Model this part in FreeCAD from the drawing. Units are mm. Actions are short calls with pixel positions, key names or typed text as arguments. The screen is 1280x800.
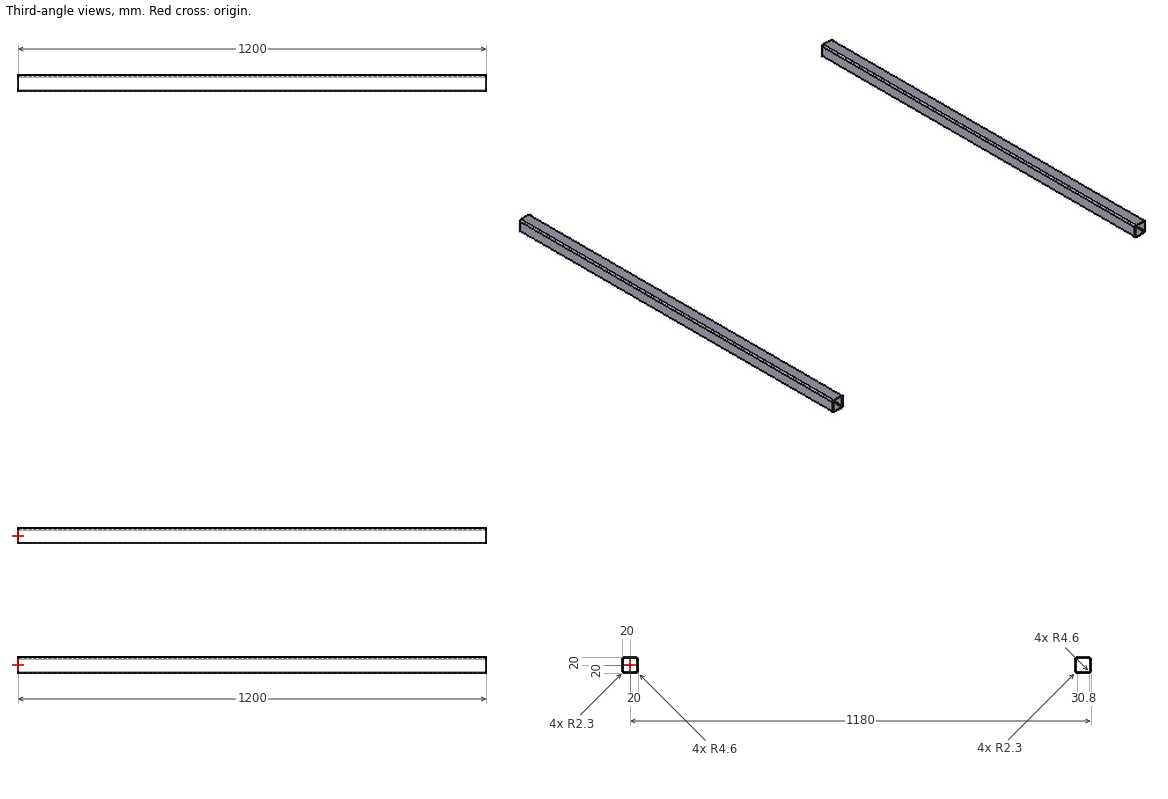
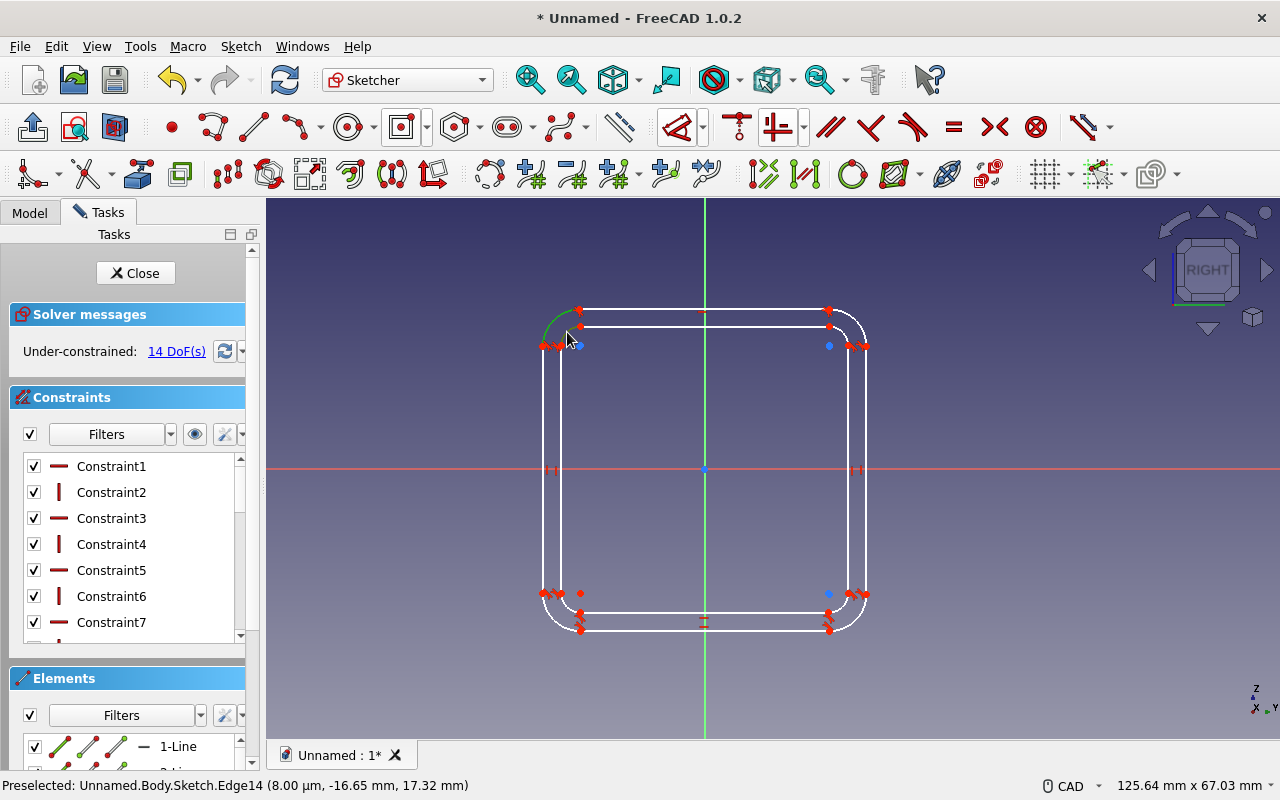
key(c)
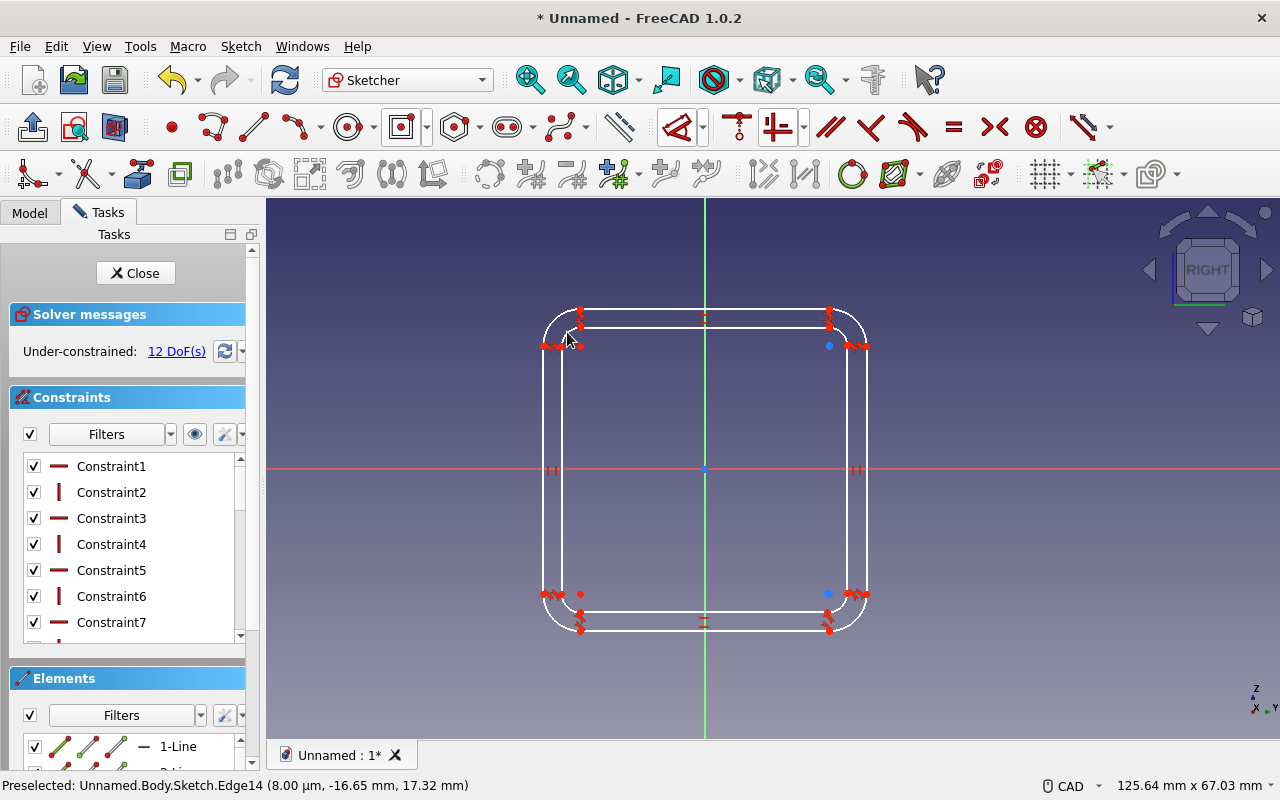
click(863, 329)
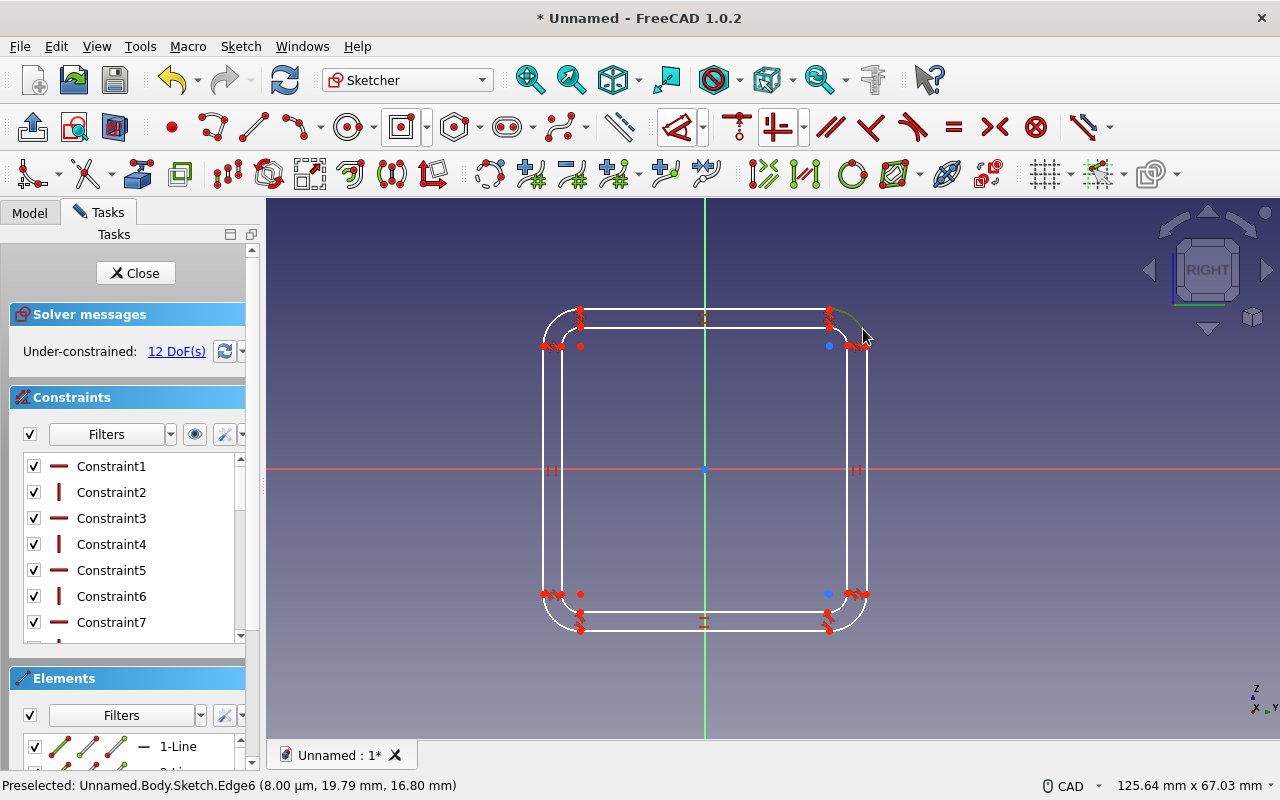
click(842, 333)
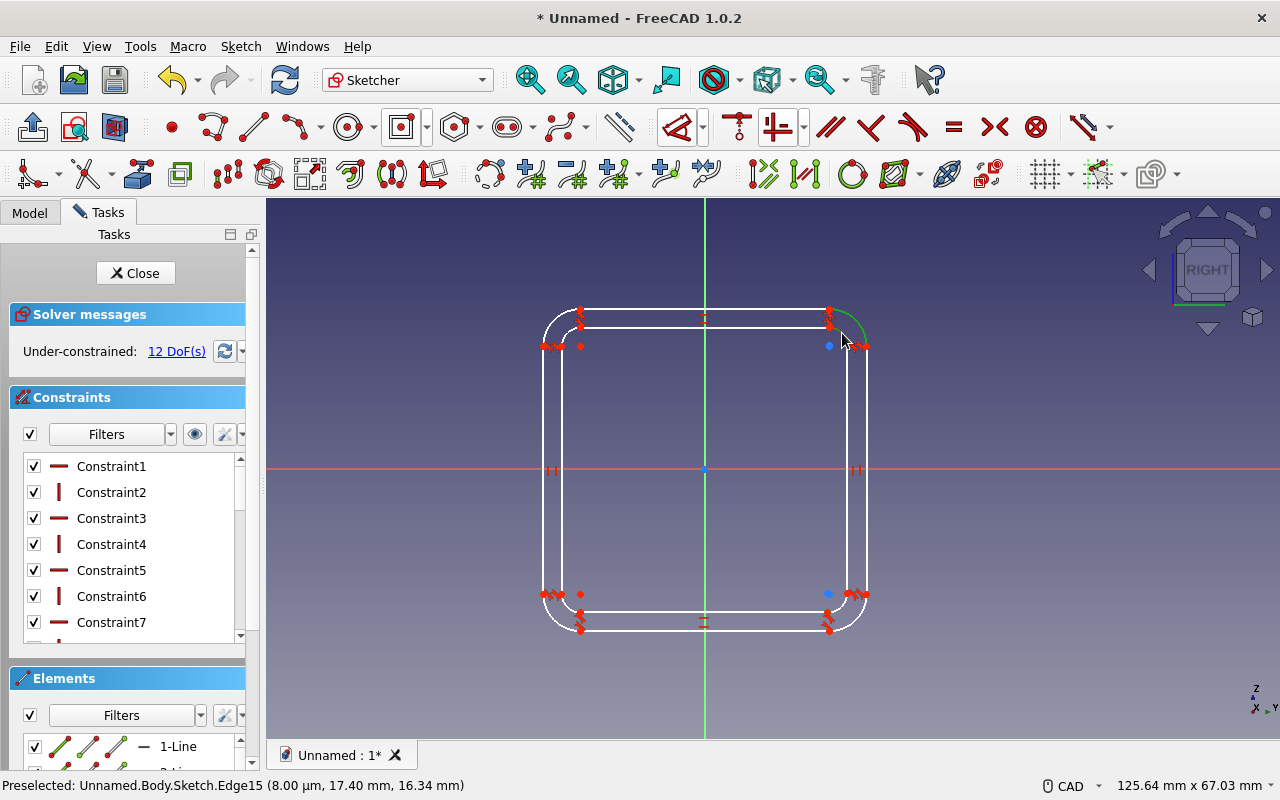
key(c)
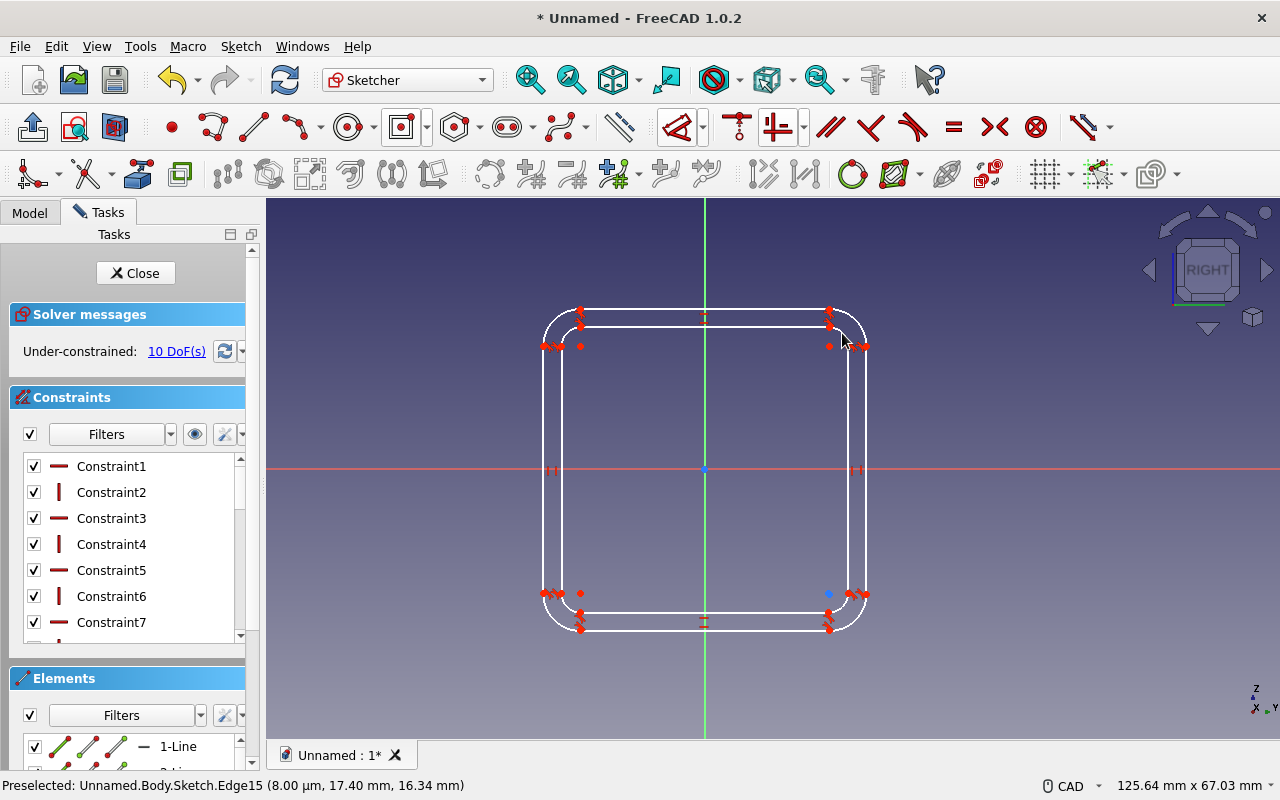
click(846, 627)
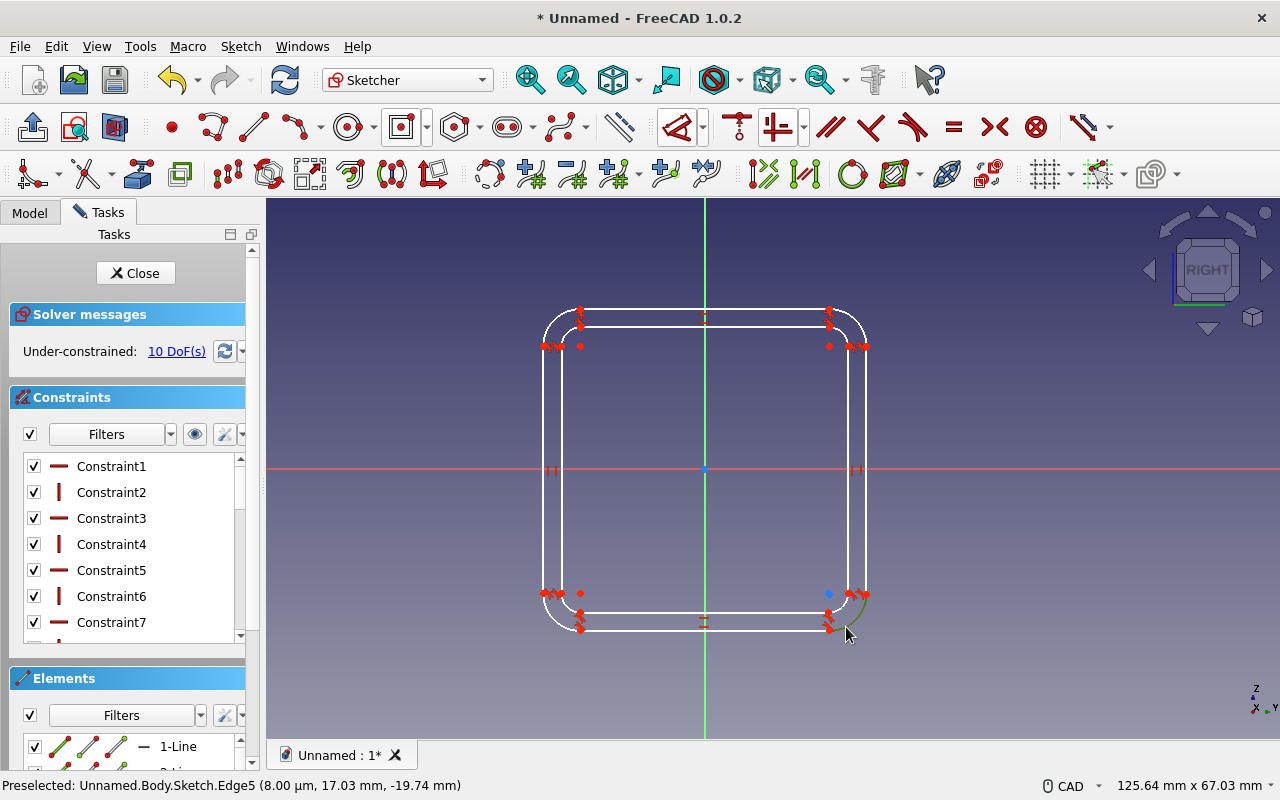
click(862, 329)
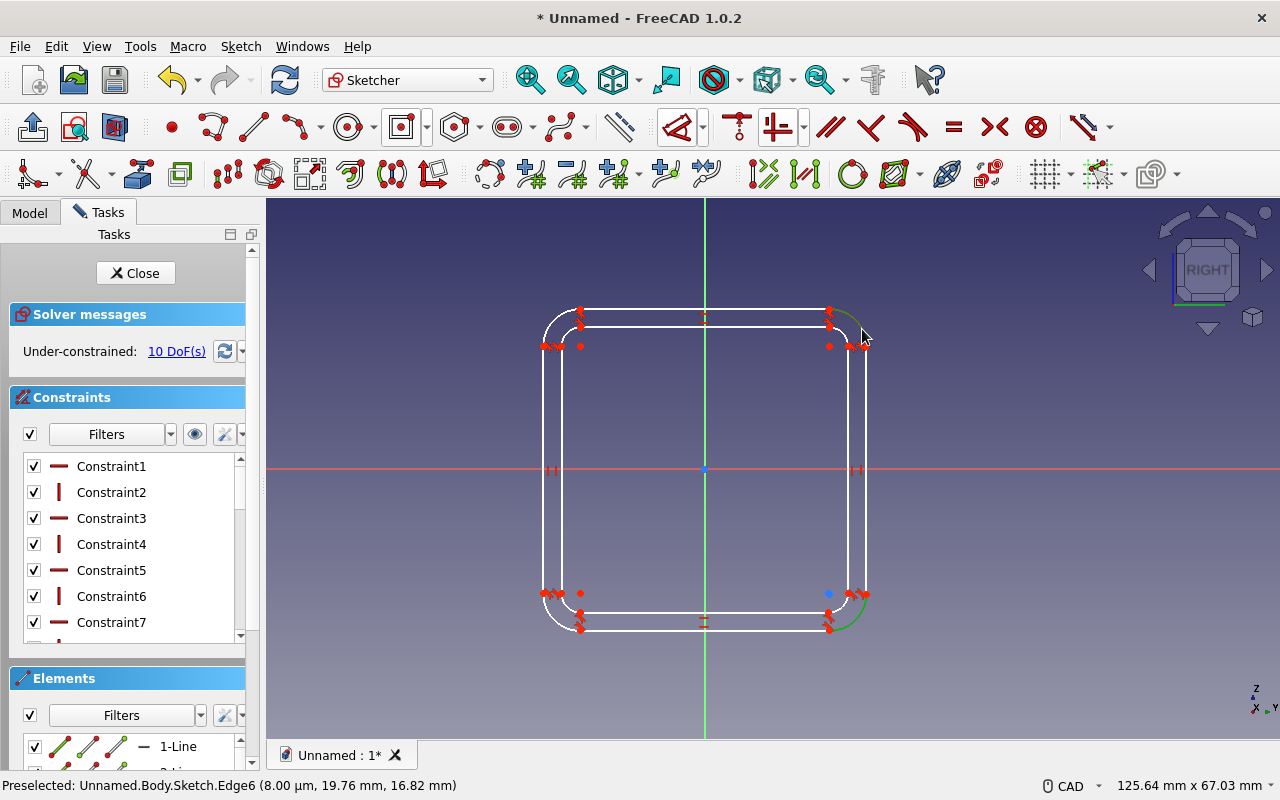
click(564, 313)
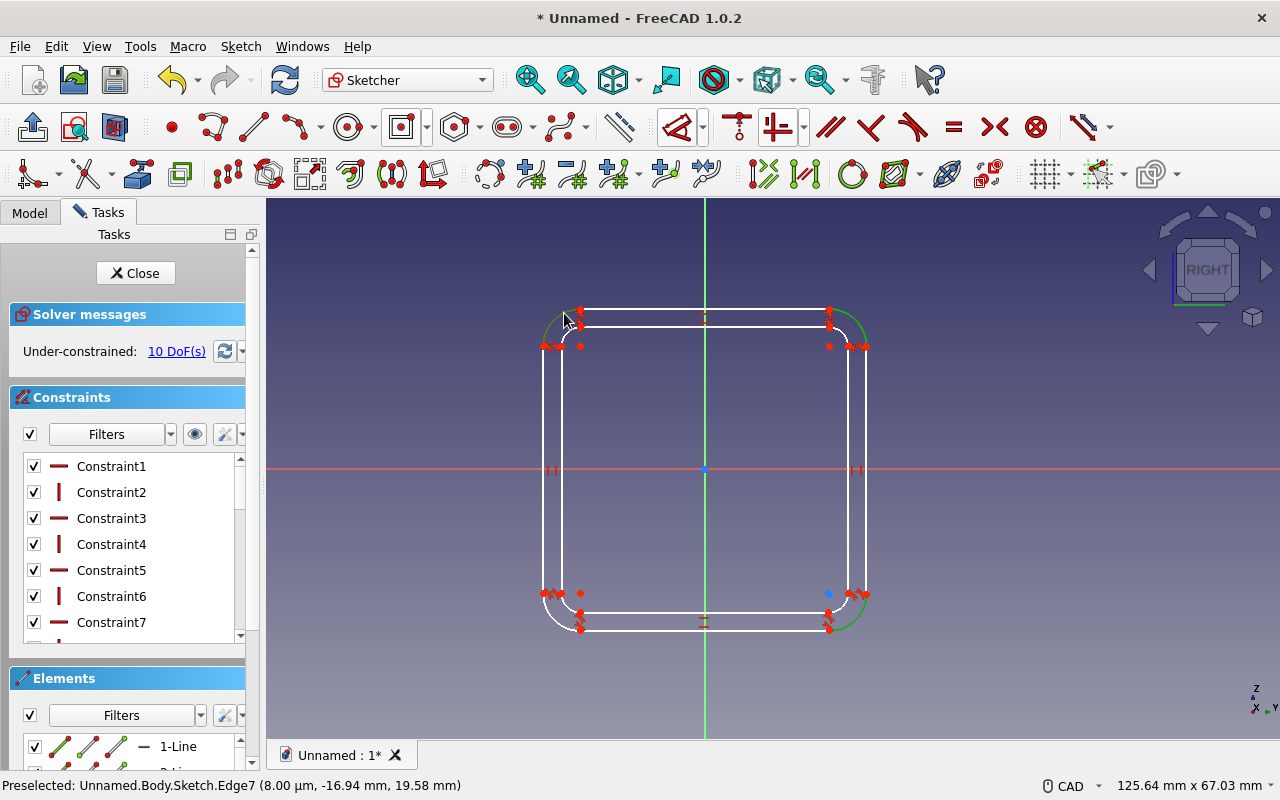
click(547, 611)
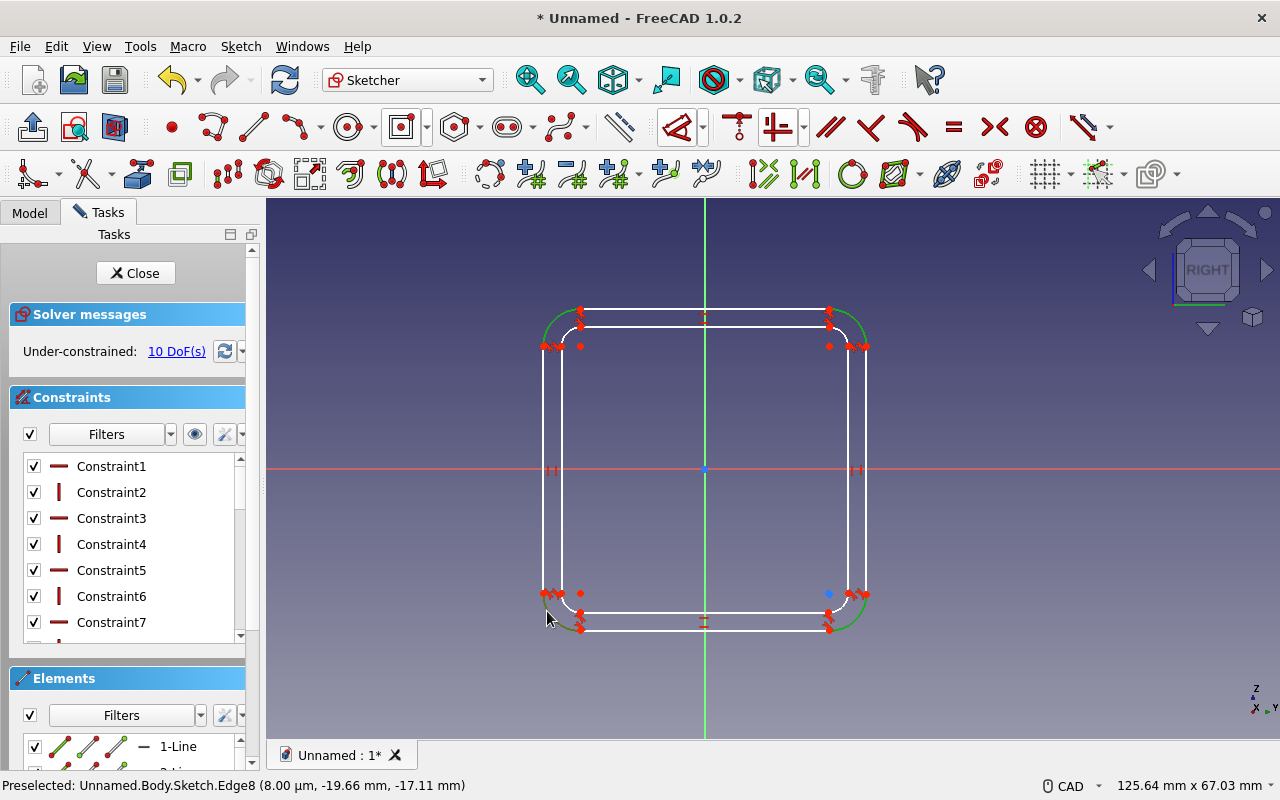
key(e)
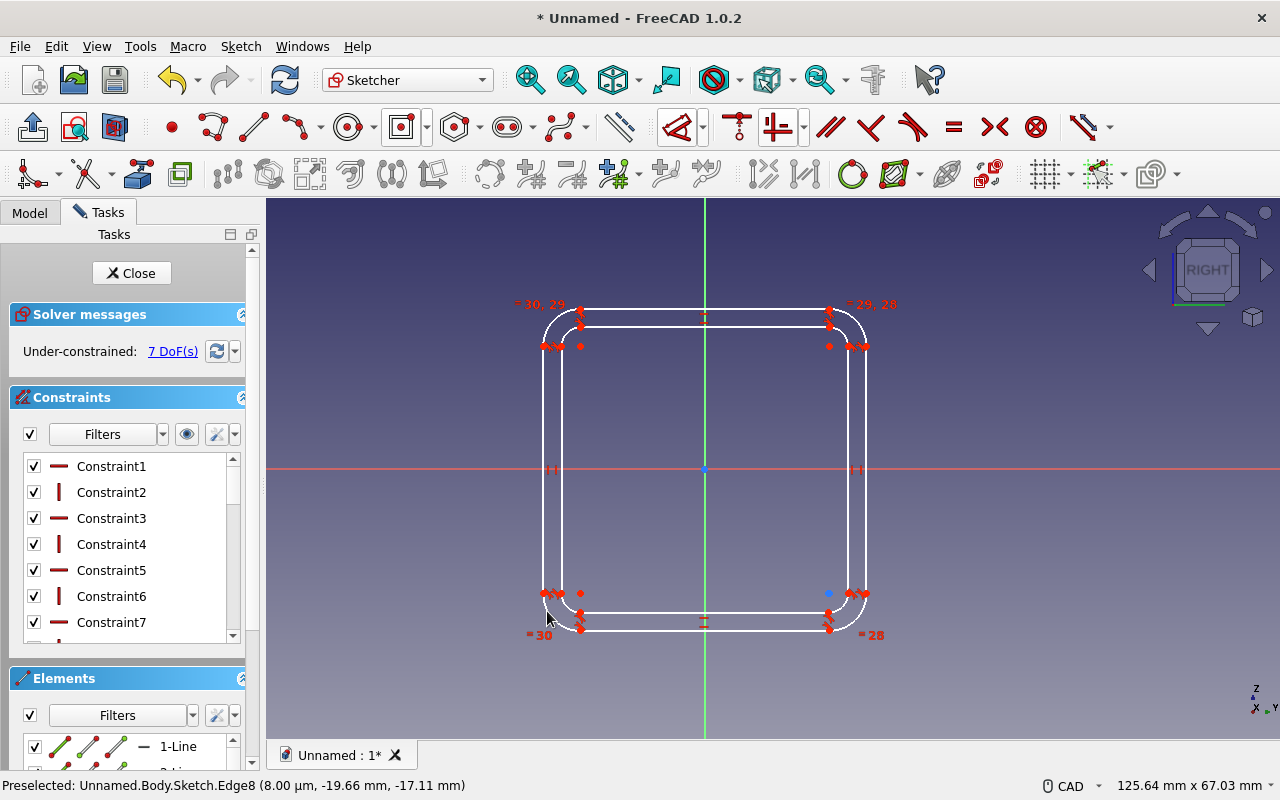
click(567, 607)